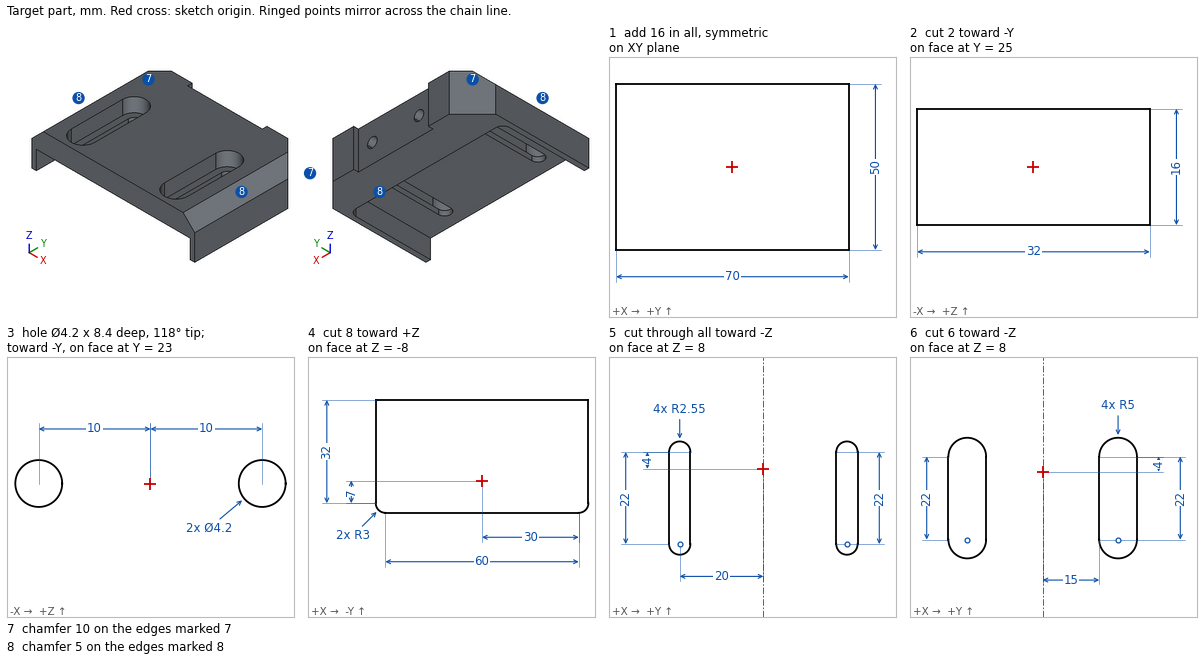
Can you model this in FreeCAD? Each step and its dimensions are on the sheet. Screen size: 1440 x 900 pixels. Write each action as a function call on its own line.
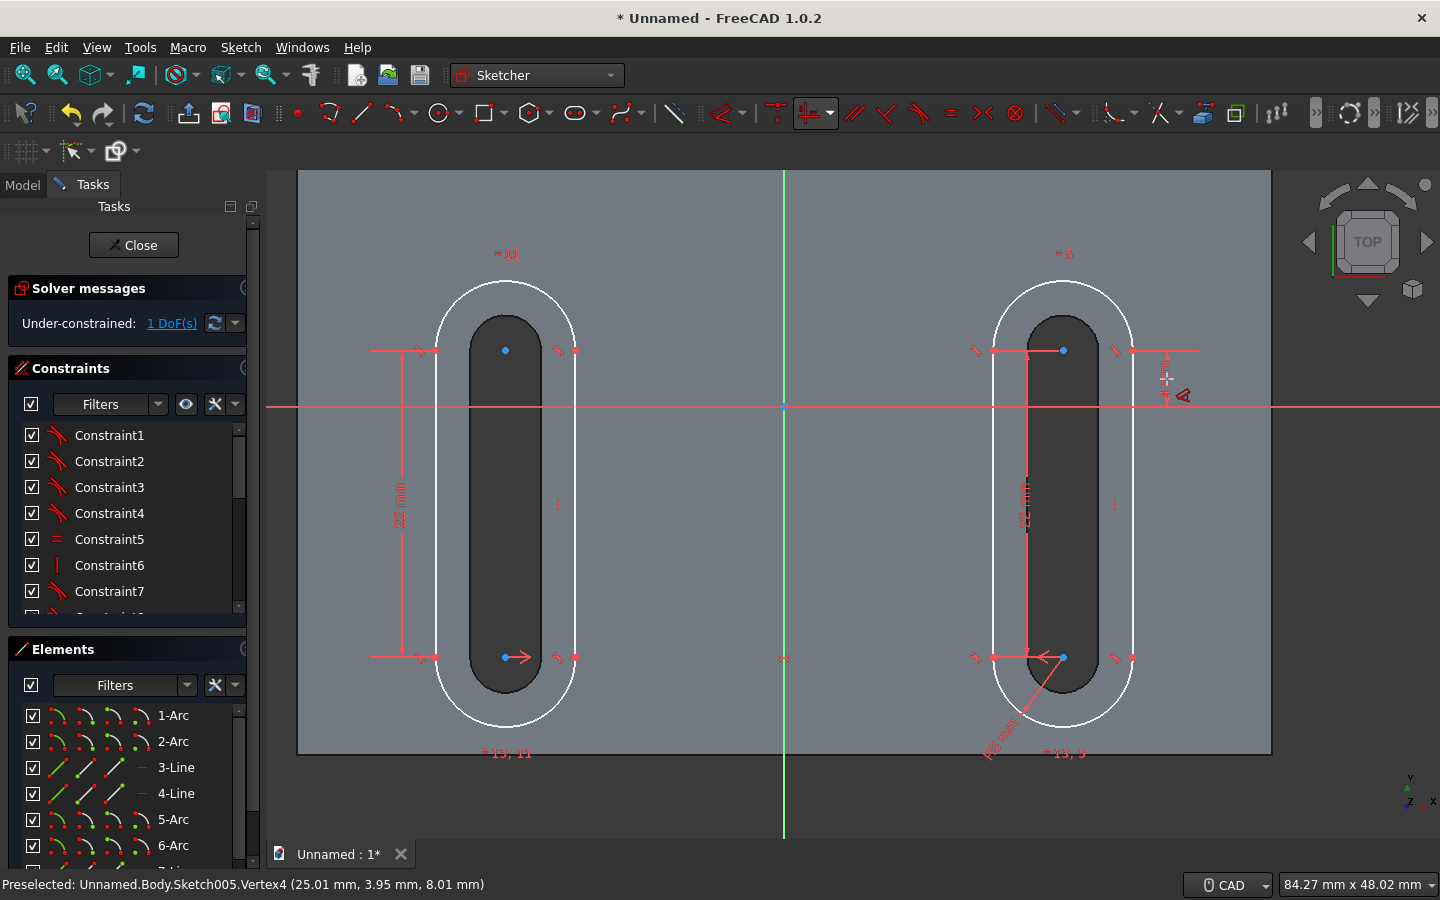
click(993, 657)
click(889, 691)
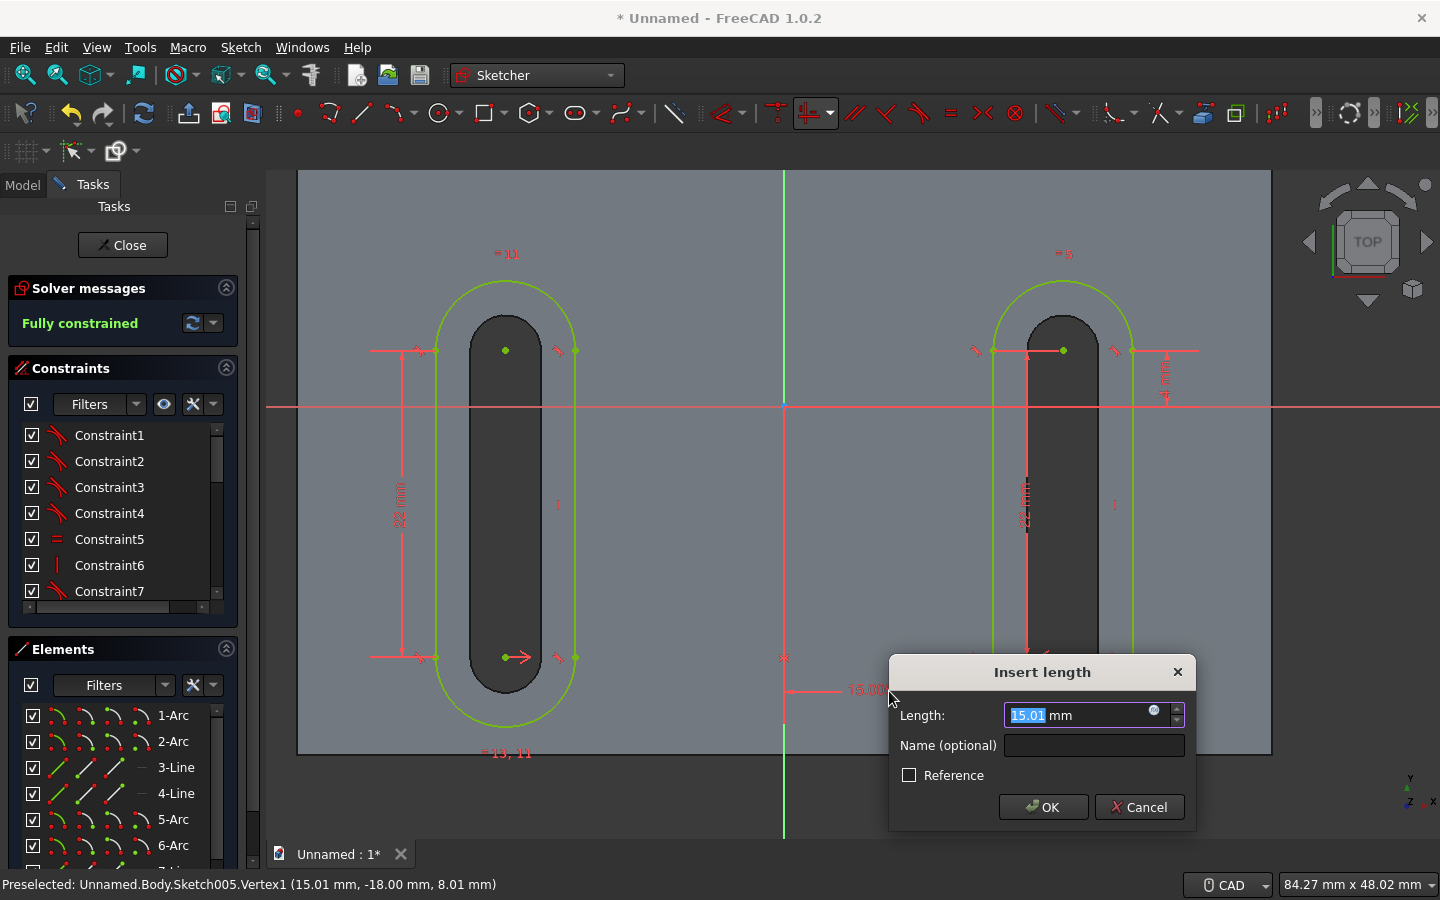
text(15)
key(Return)
key(Escape)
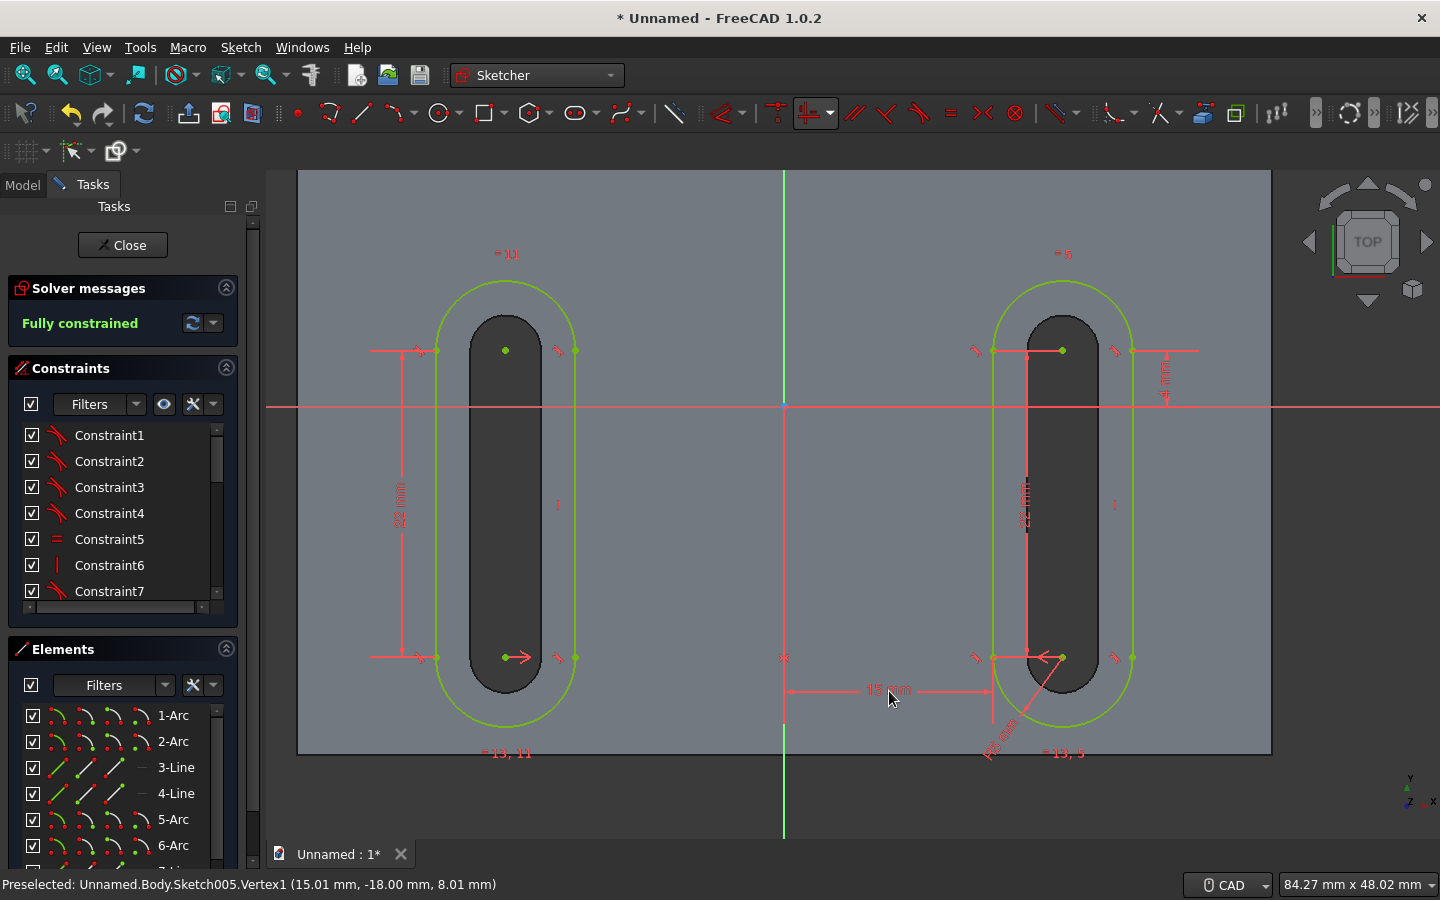
click(123, 245)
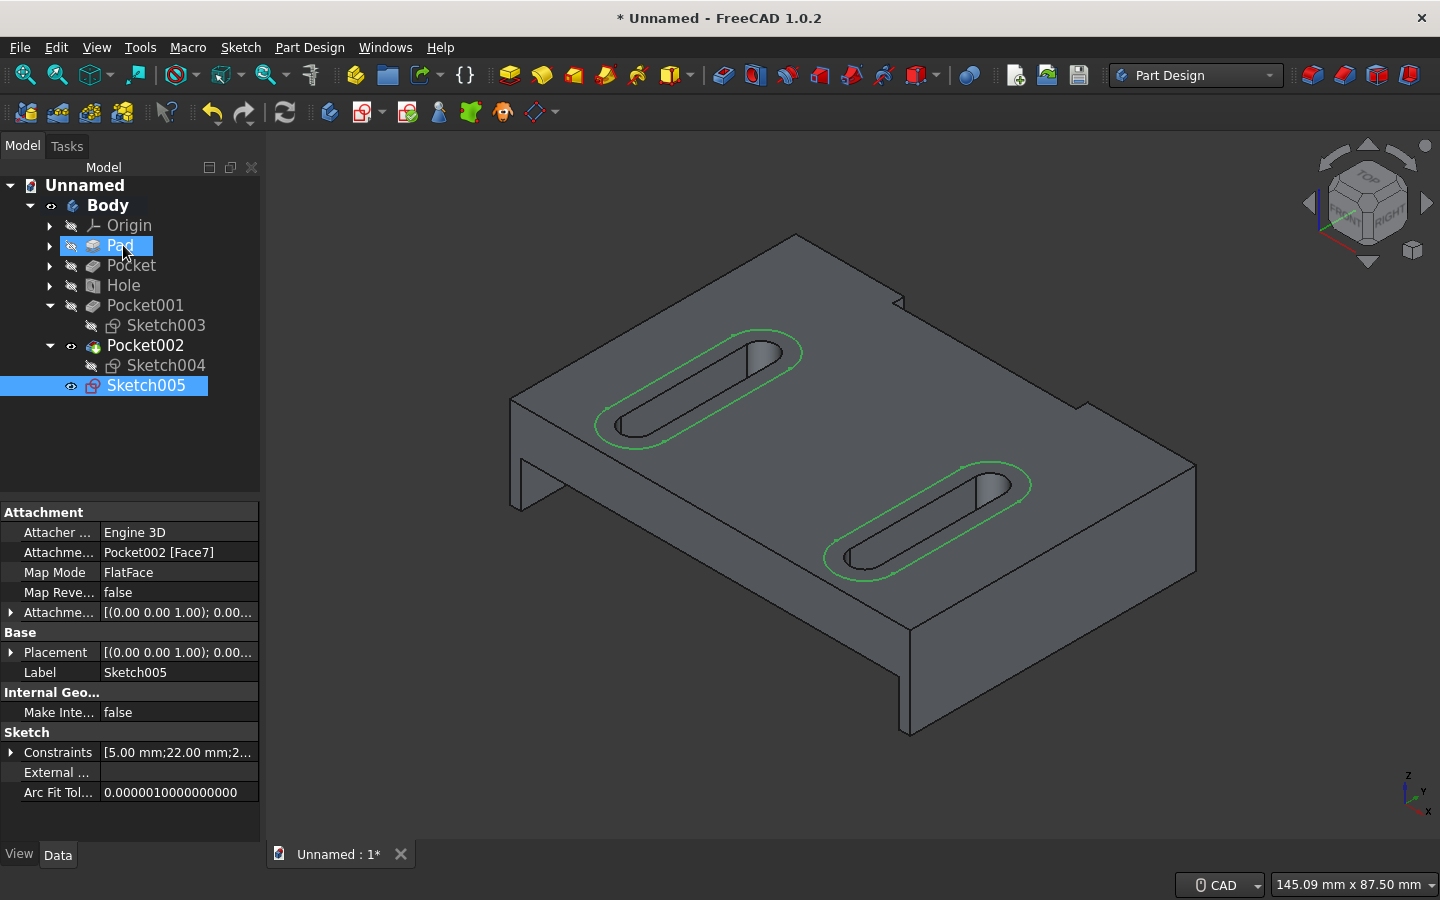
click(724, 76)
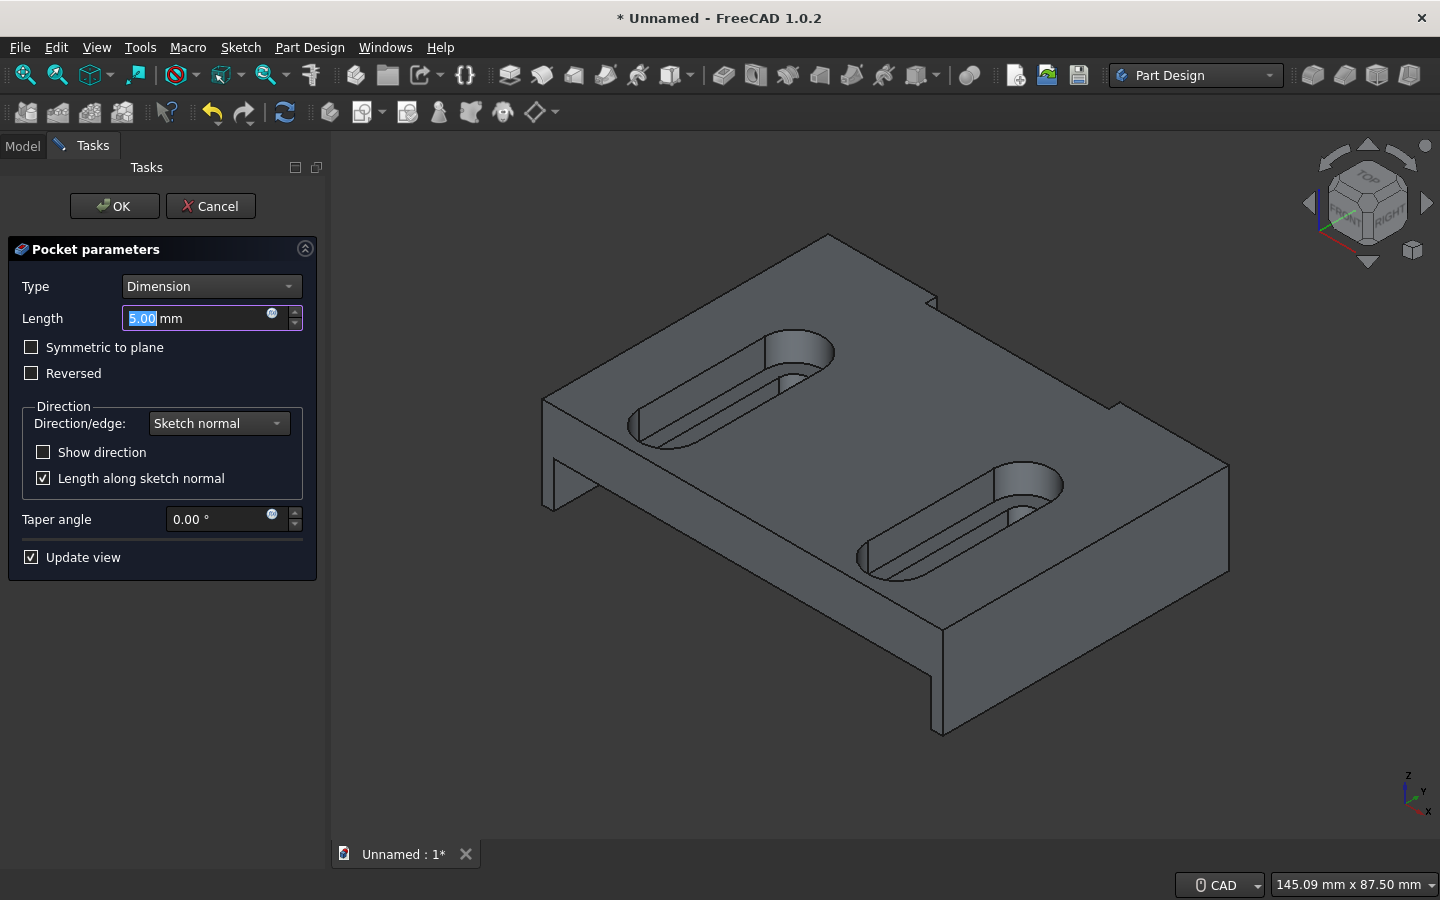
text(6)
key(Tab)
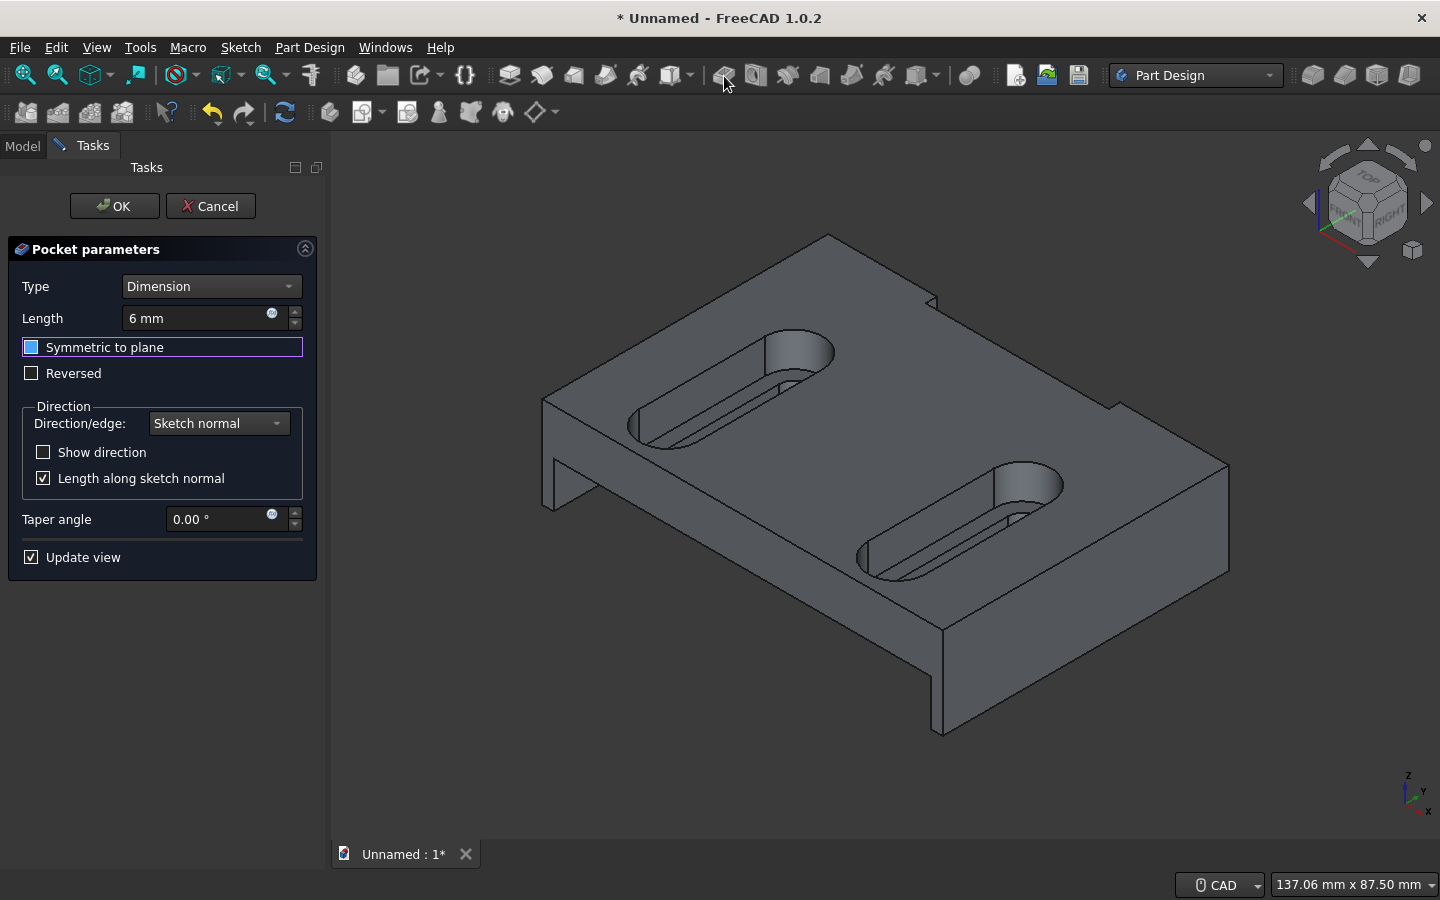
click(115, 206)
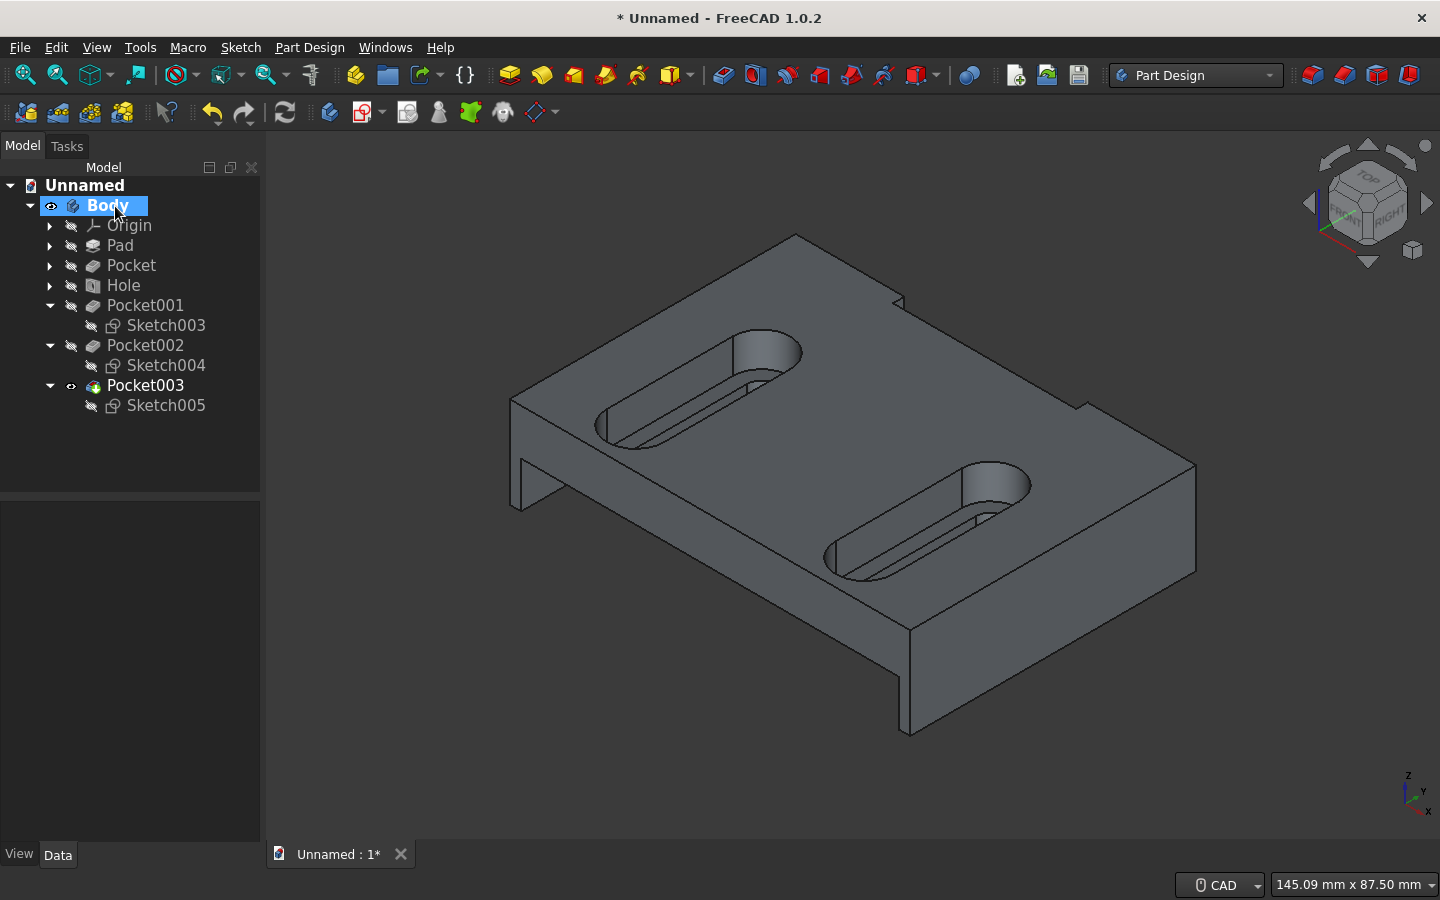
key(2)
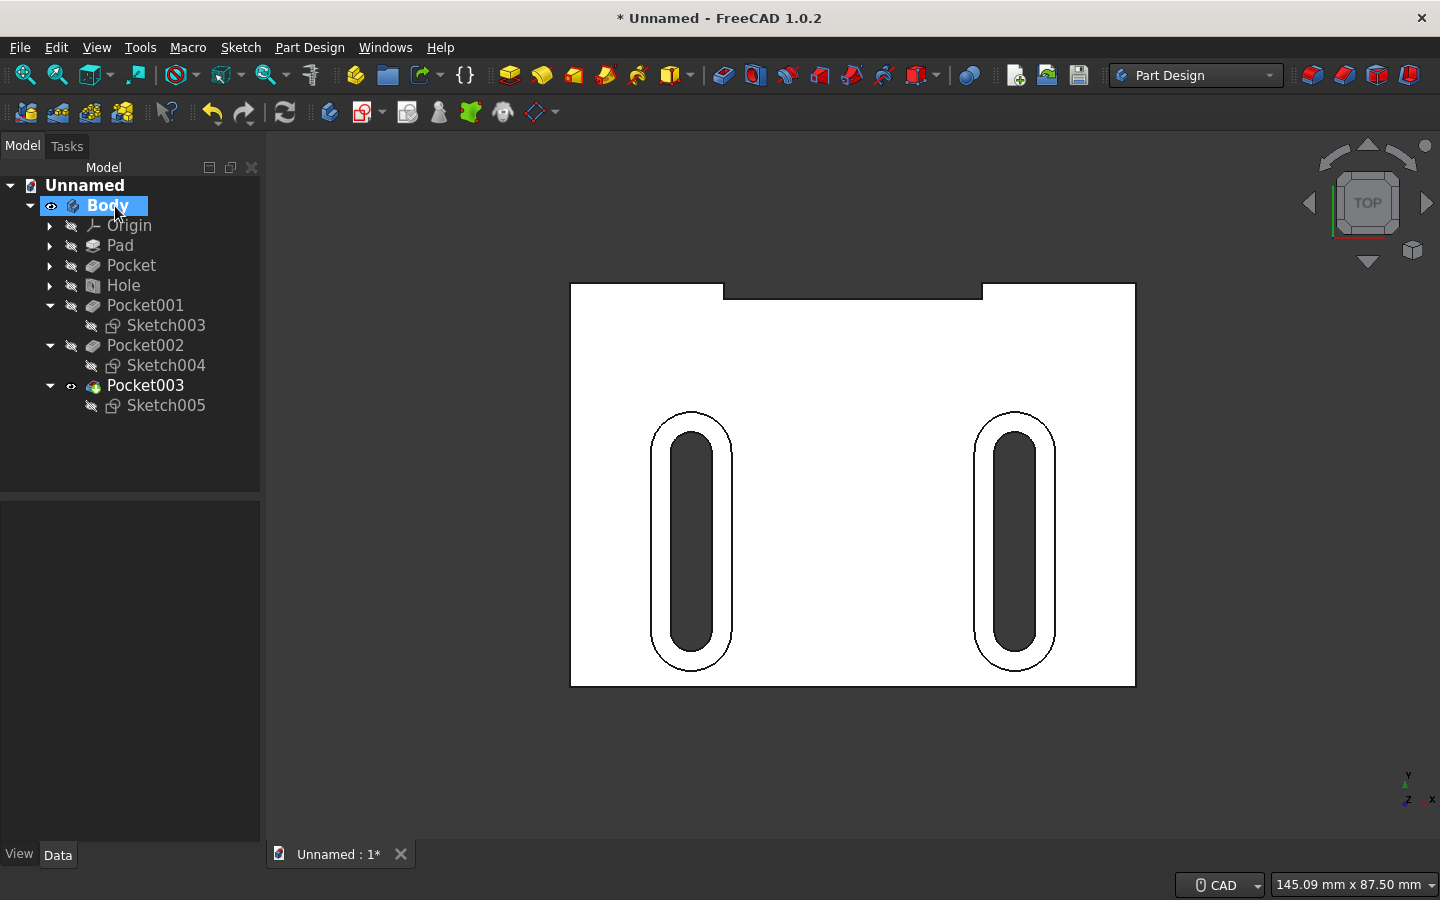
key(0)